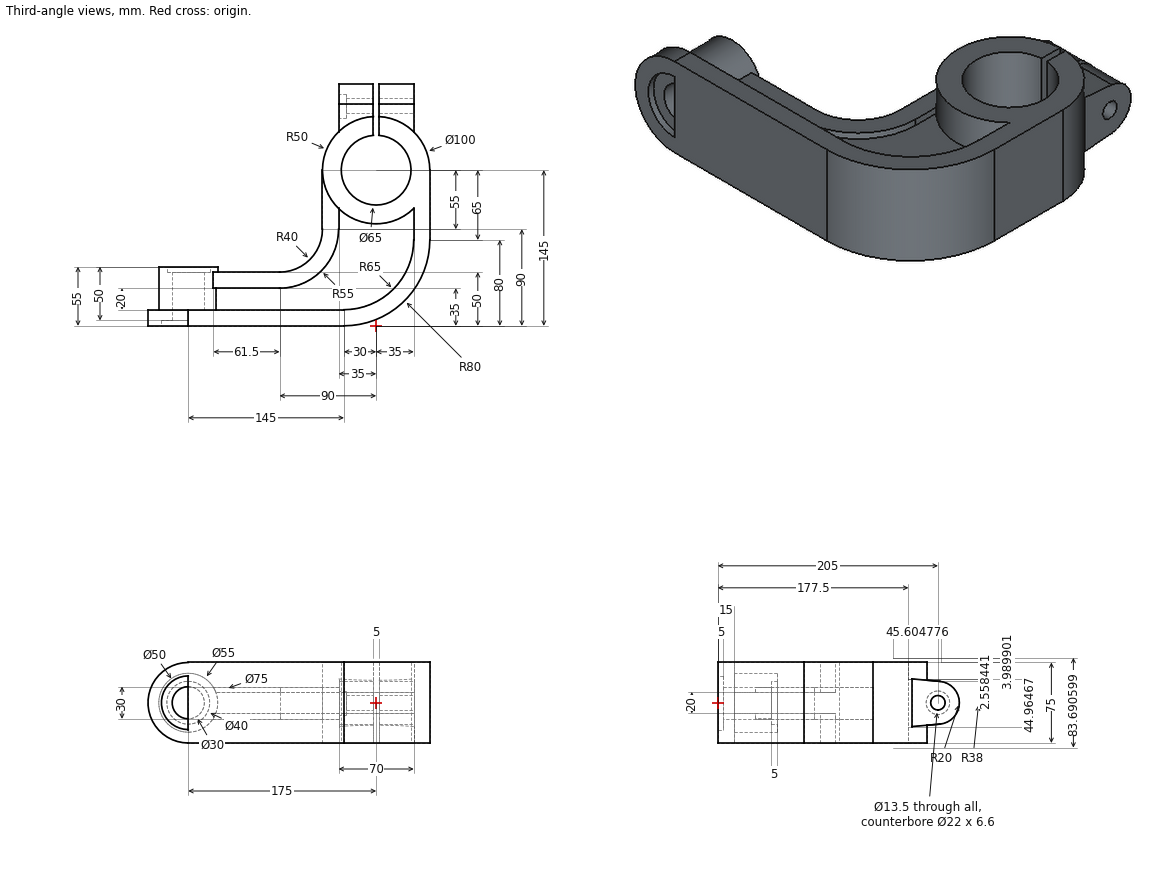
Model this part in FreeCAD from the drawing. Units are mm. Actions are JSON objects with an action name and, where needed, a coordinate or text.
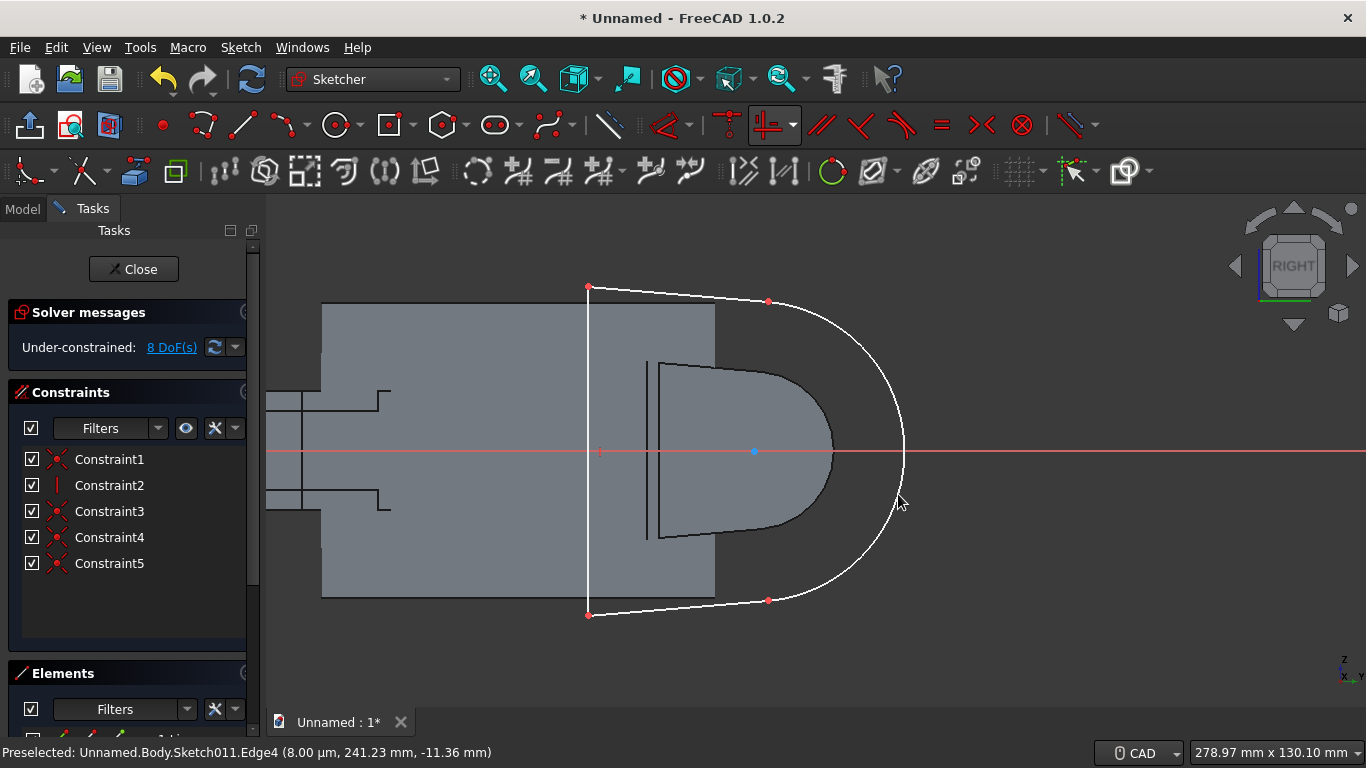
{"action": "left_click", "coordinate": [714, 297]}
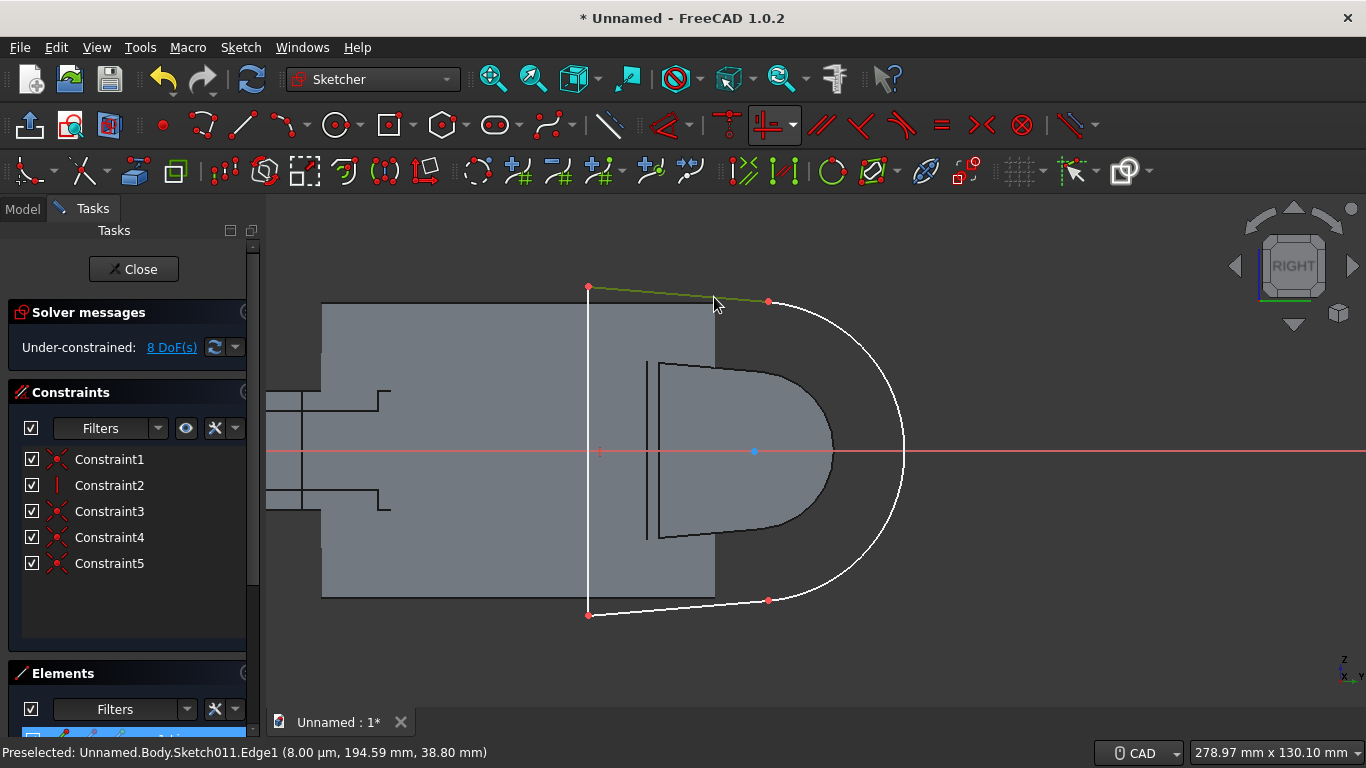
{"action": "left_click", "coordinate": [879, 535]}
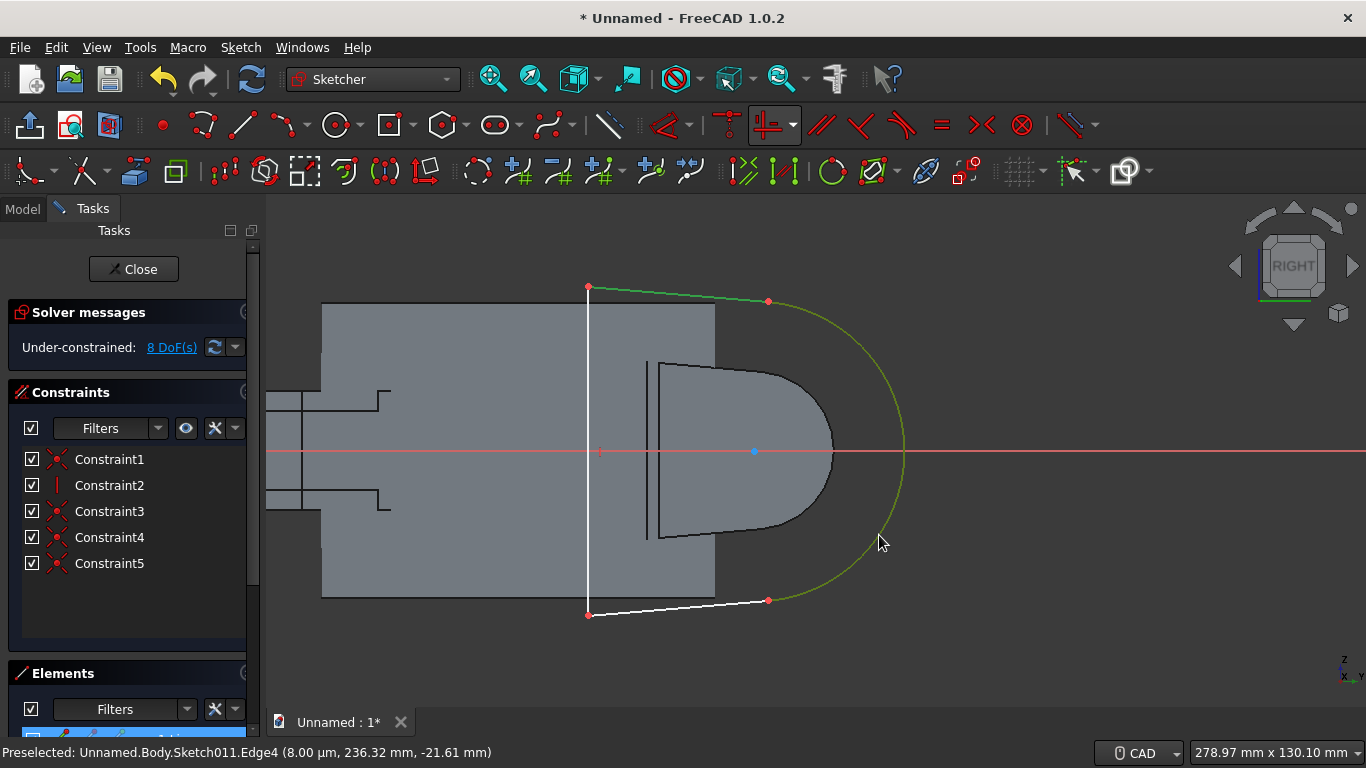
{"action": "key", "text": "t"}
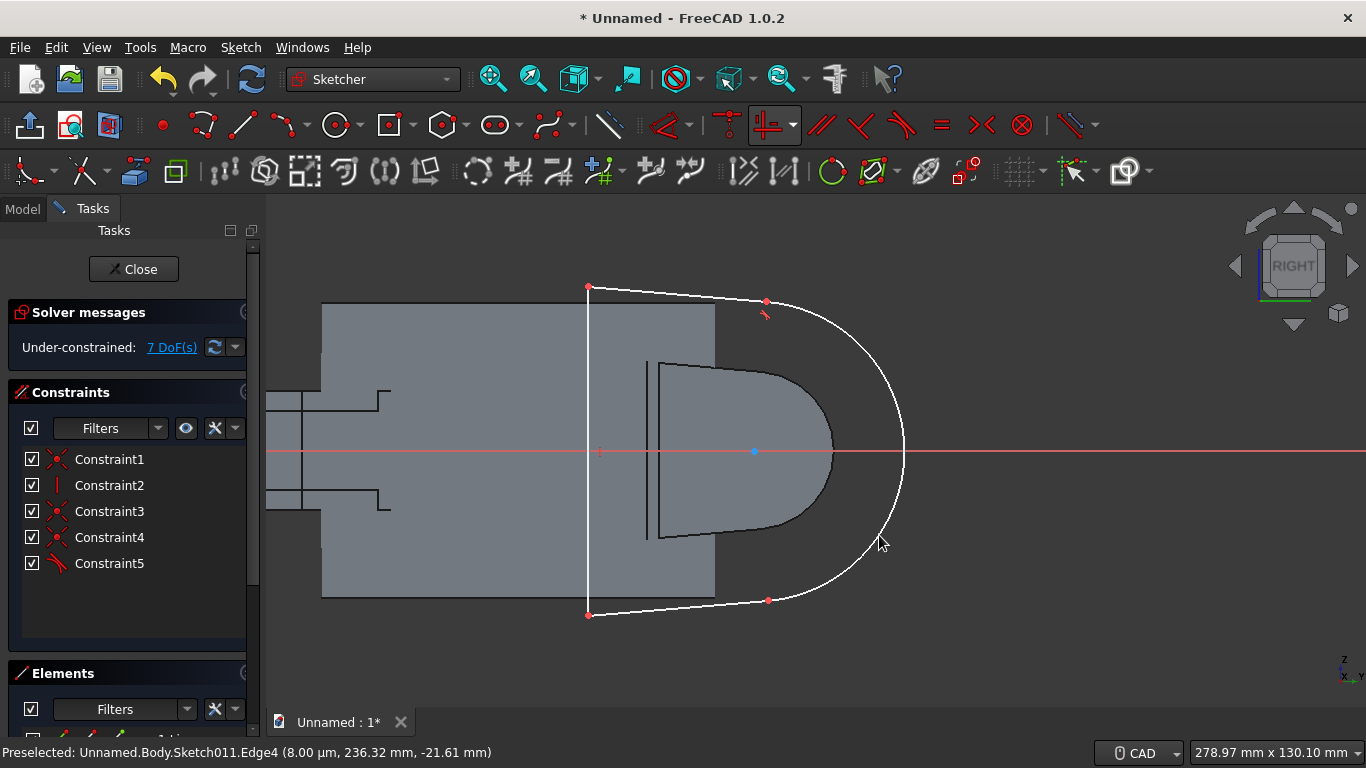
{"action": "left_click", "coordinate": [642, 612]}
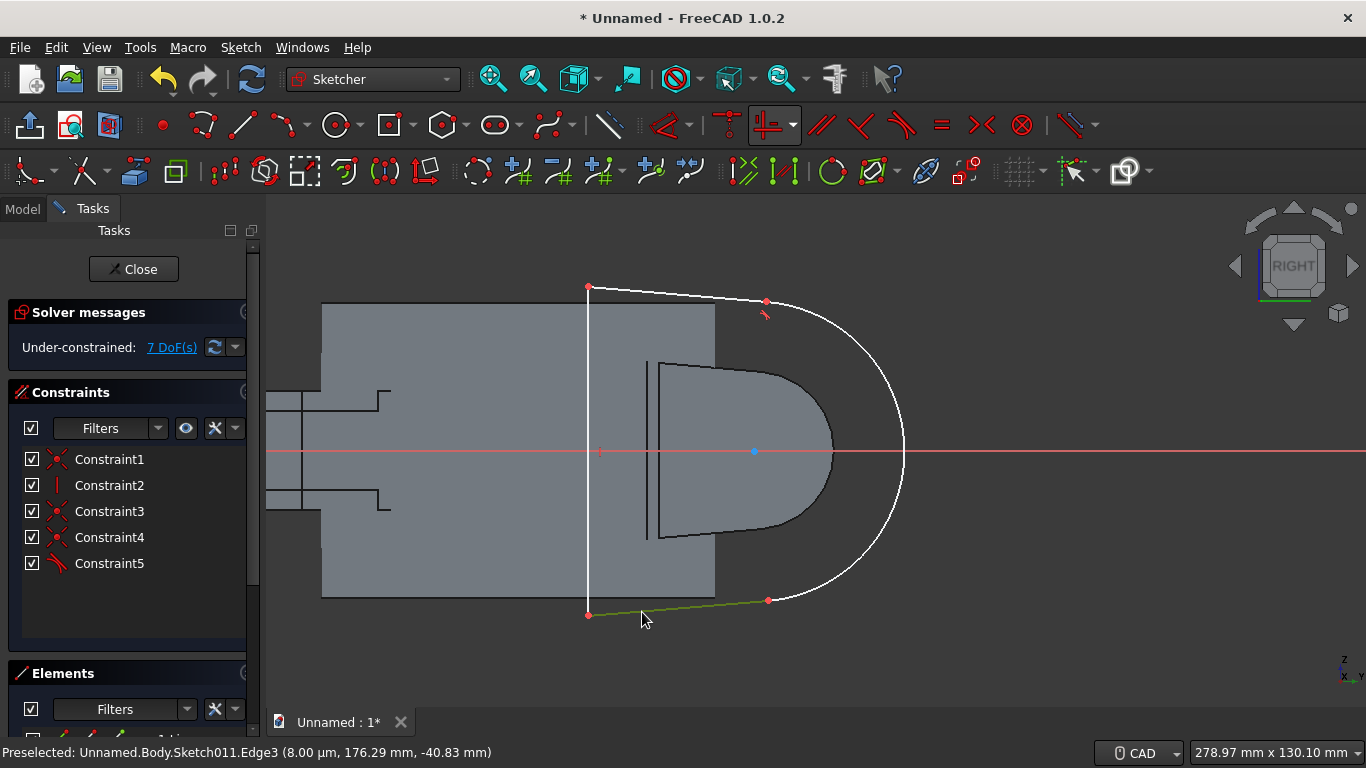
{"action": "left_click", "coordinate": [879, 535]}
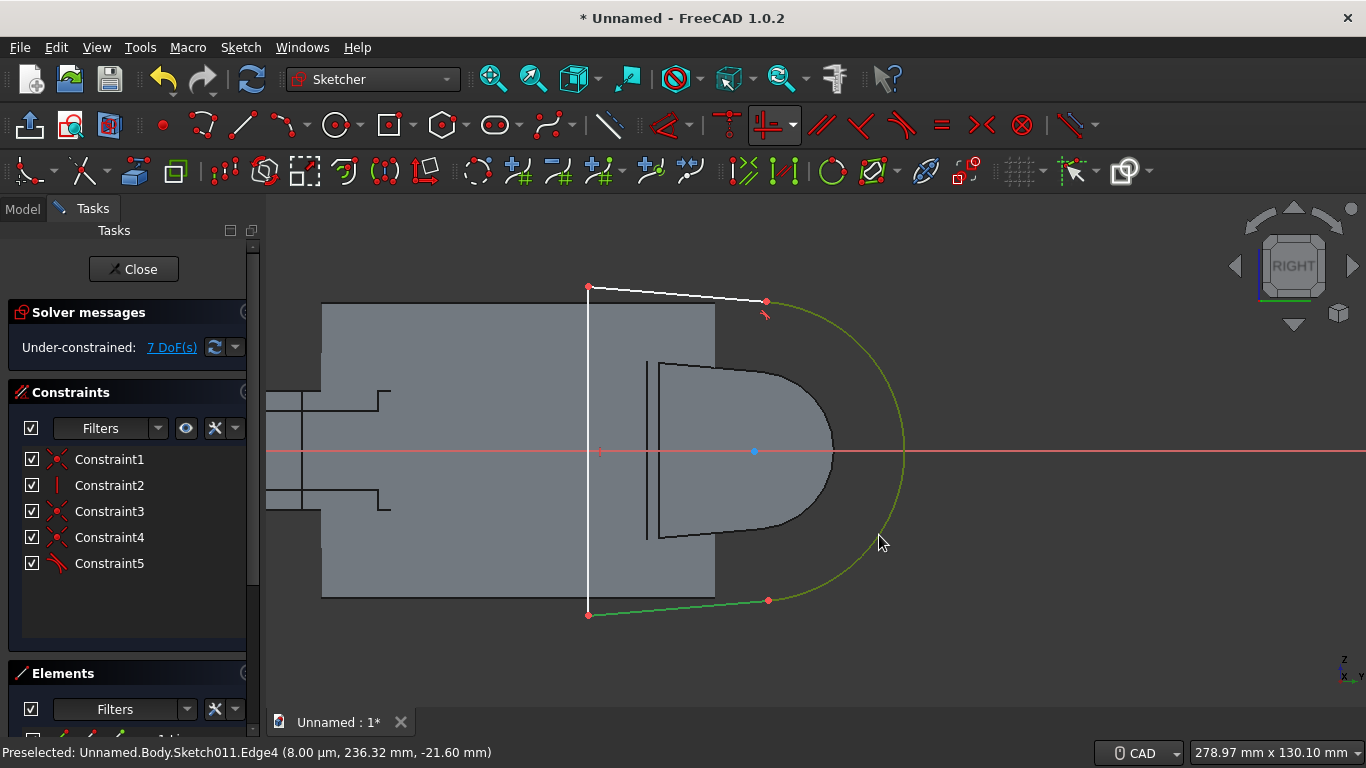
{"action": "key", "text": "t"}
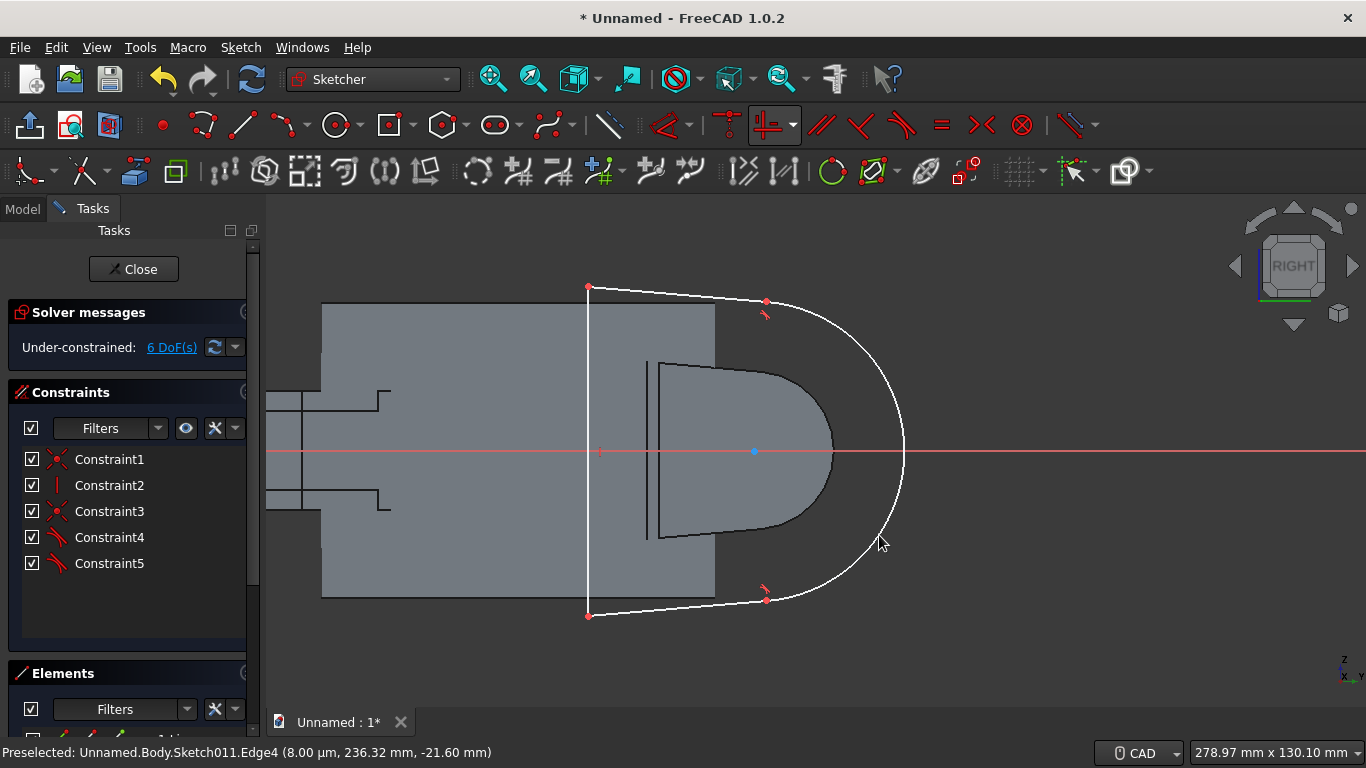
{"action": "left_click", "coordinate": [754, 451]}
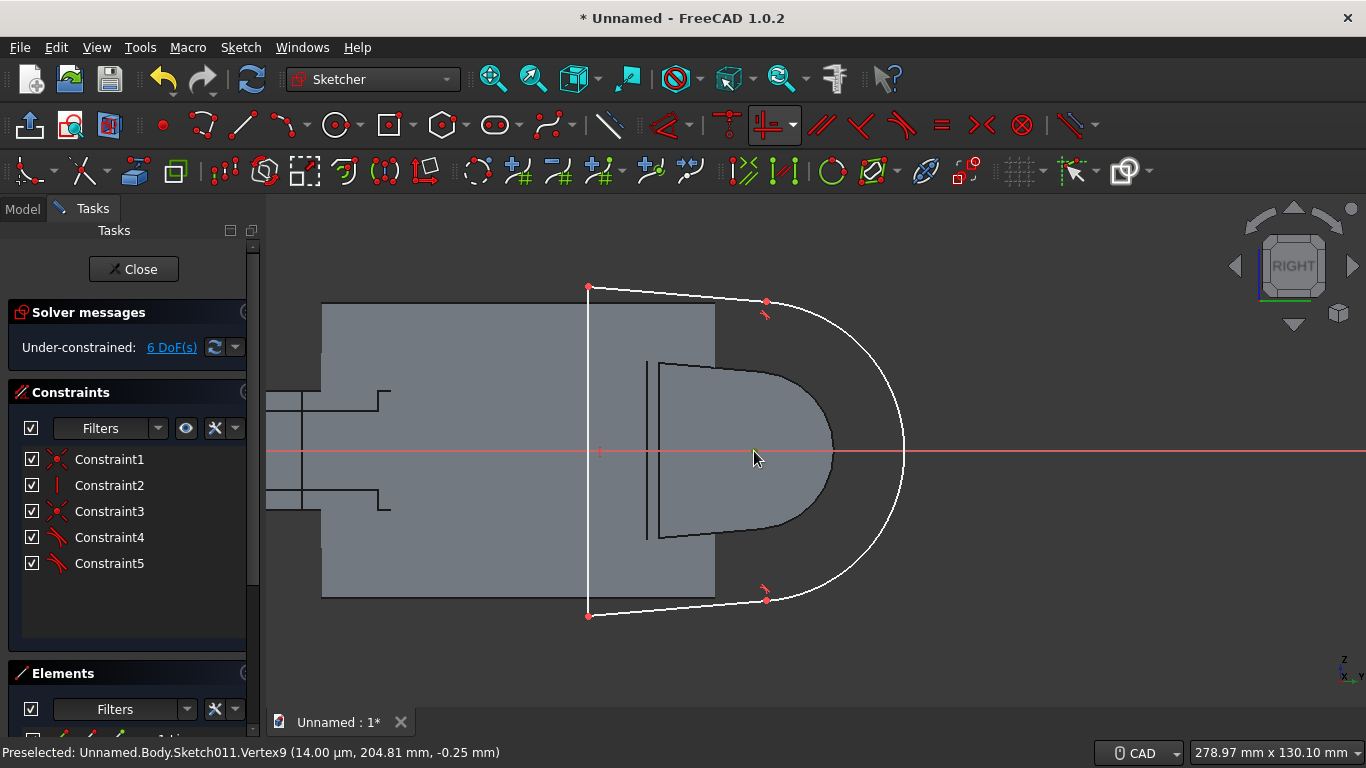
{"action": "left_click", "coordinate": [359, 450]}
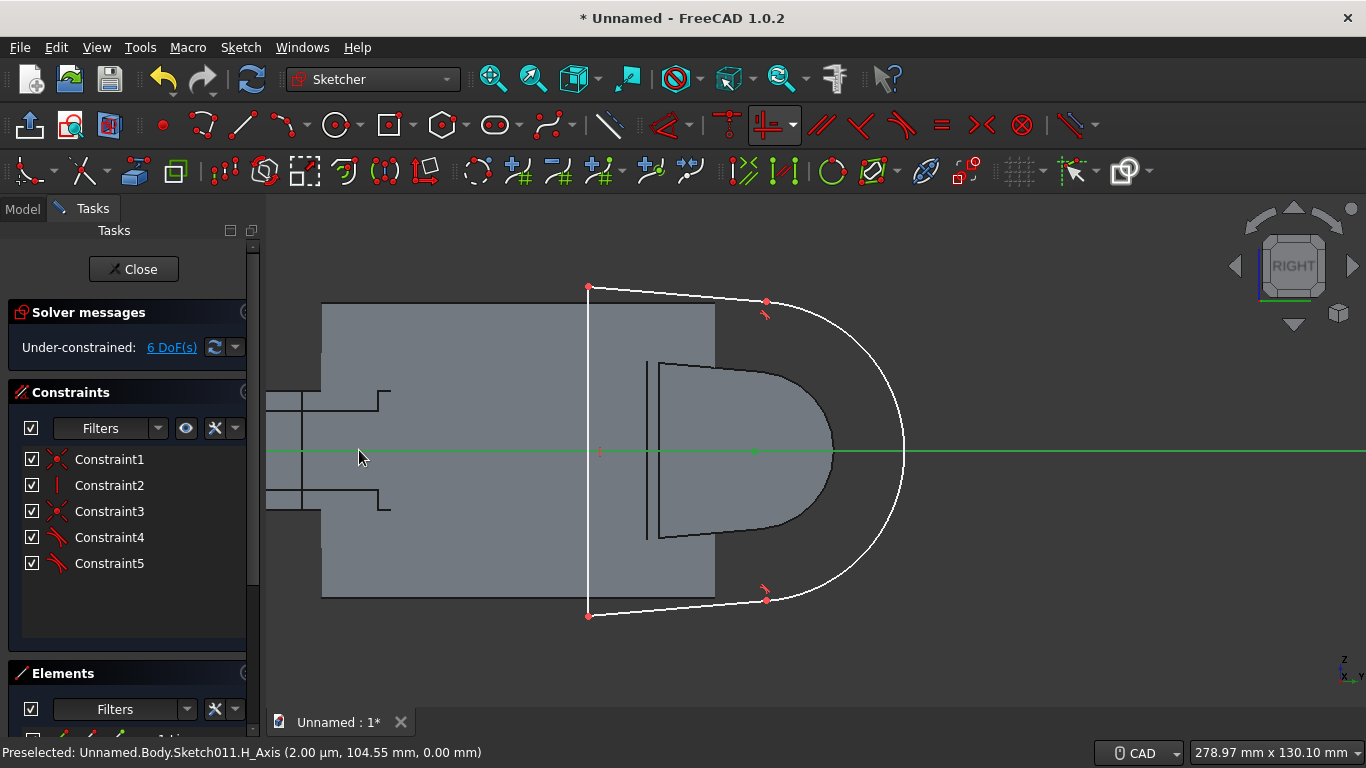
{"action": "left_click", "coordinate": [728, 126]}